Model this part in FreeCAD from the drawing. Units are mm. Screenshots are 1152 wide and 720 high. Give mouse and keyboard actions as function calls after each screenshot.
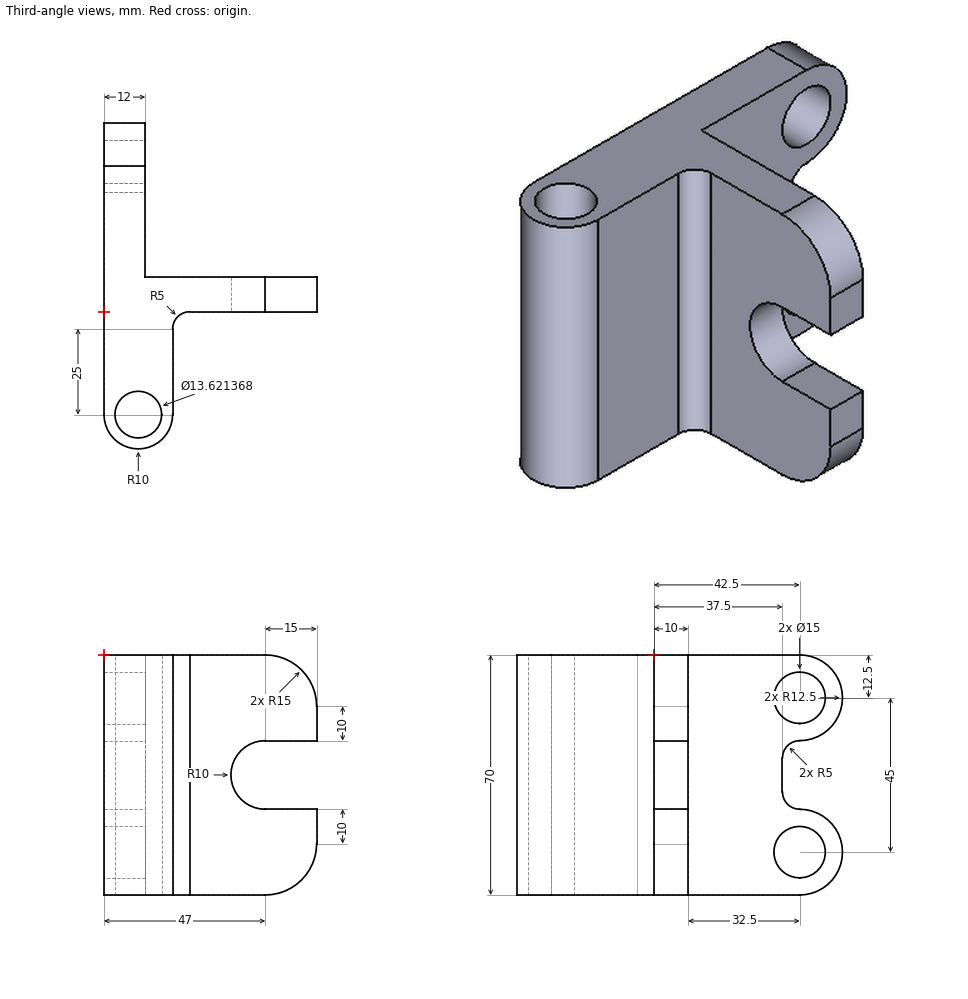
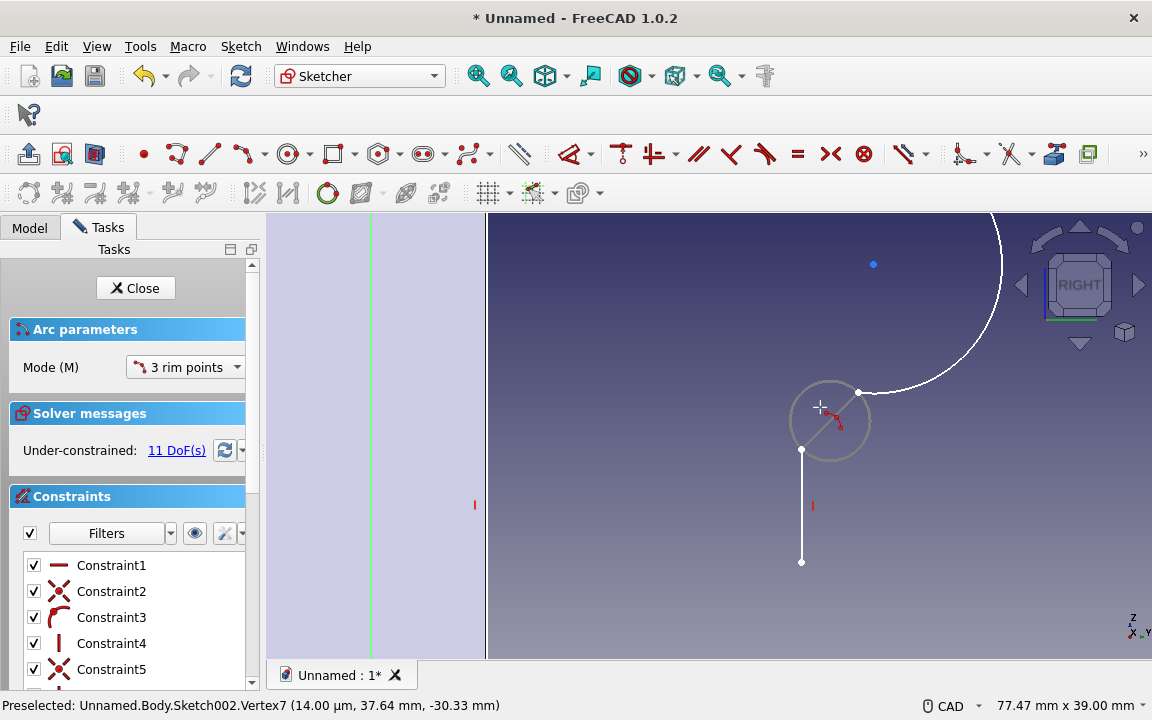
click(817, 405)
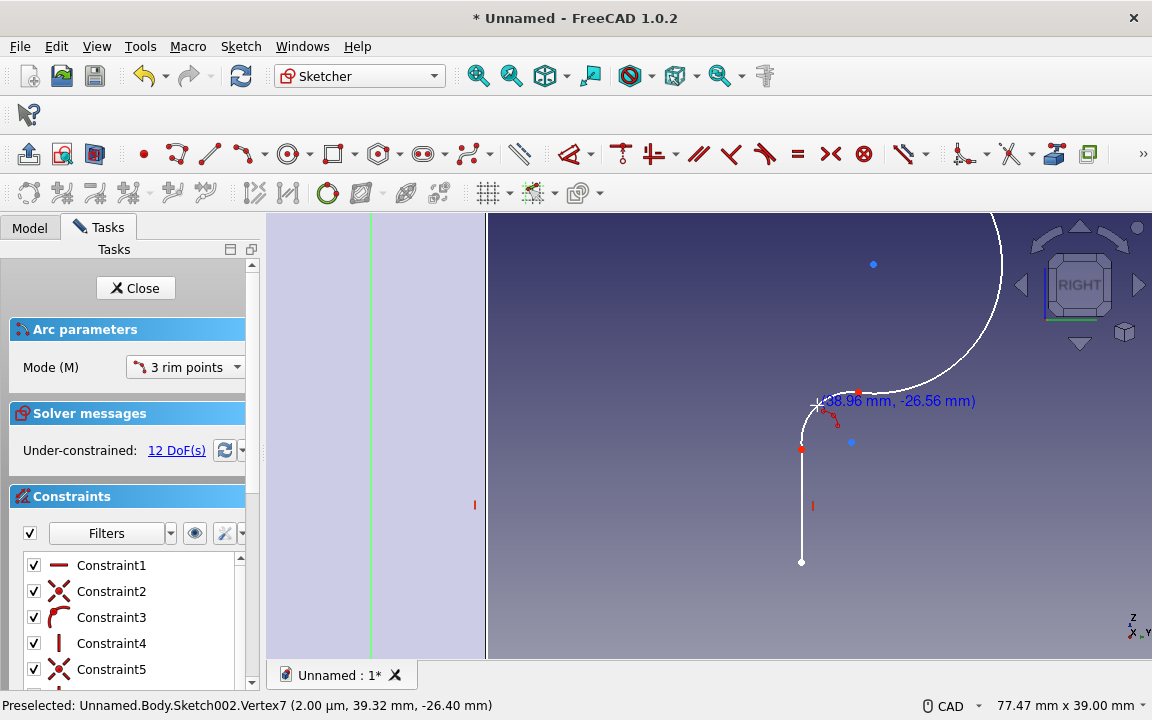
click(802, 562)
click(858, 617)
click(817, 600)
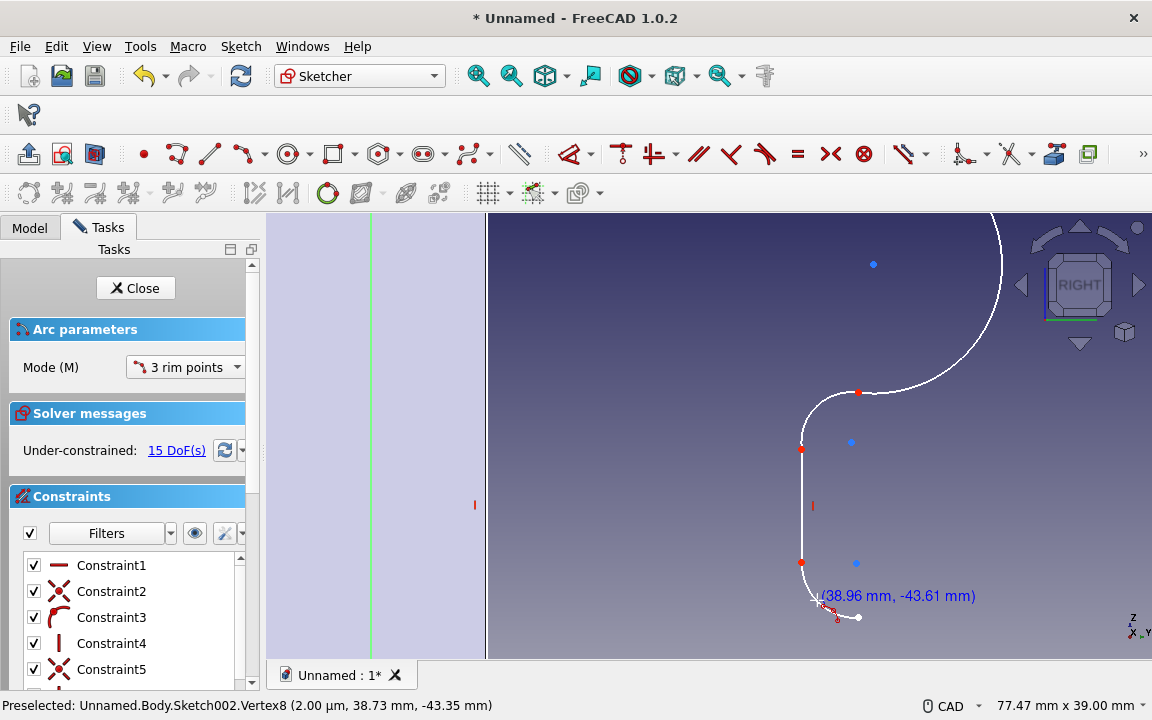
click(858, 618)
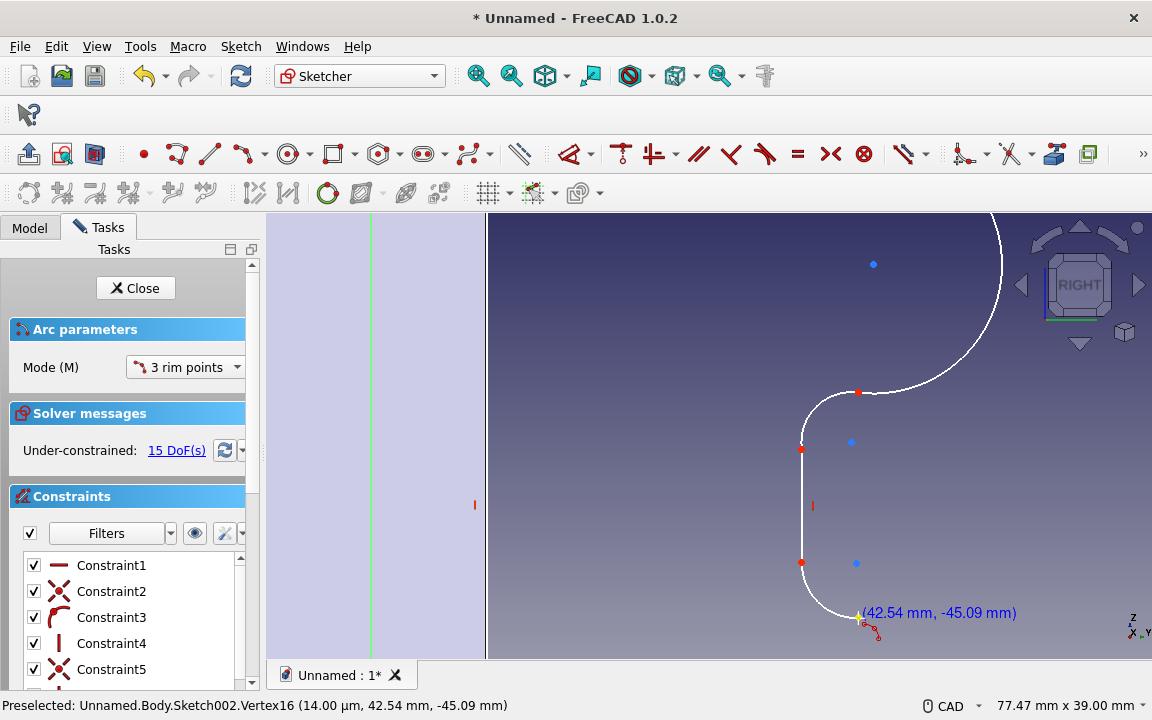
scroll(614, 397, down, 5)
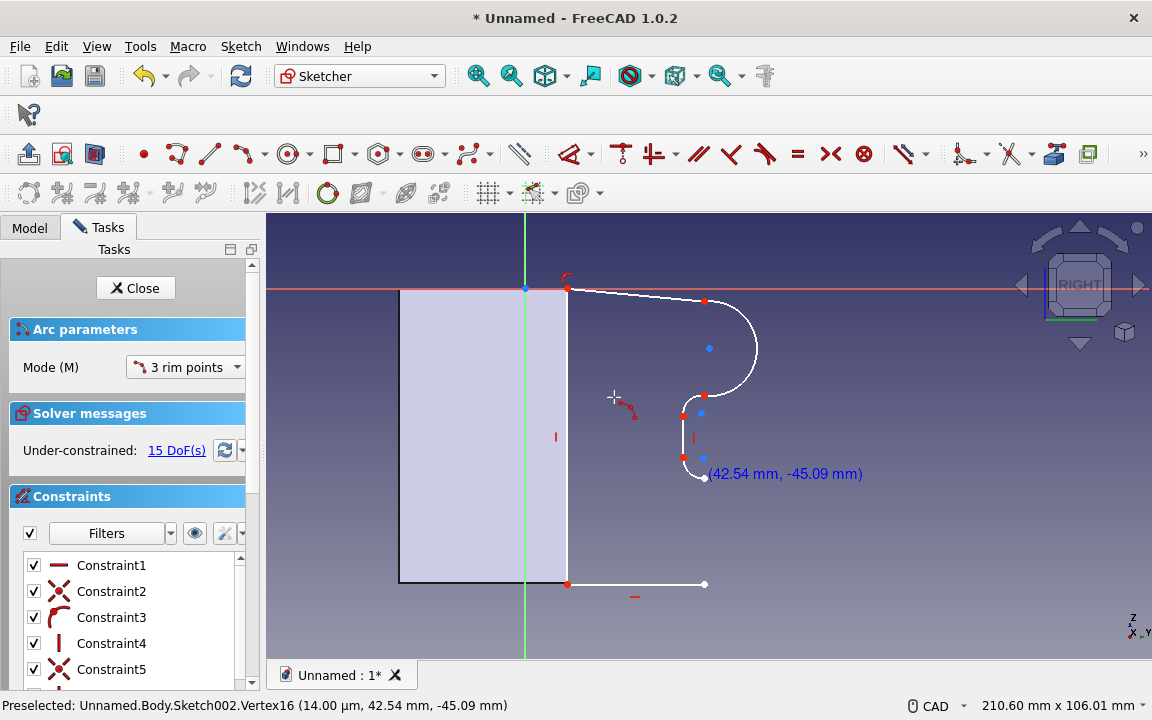
click(704, 585)
click(756, 531)
key(Escape)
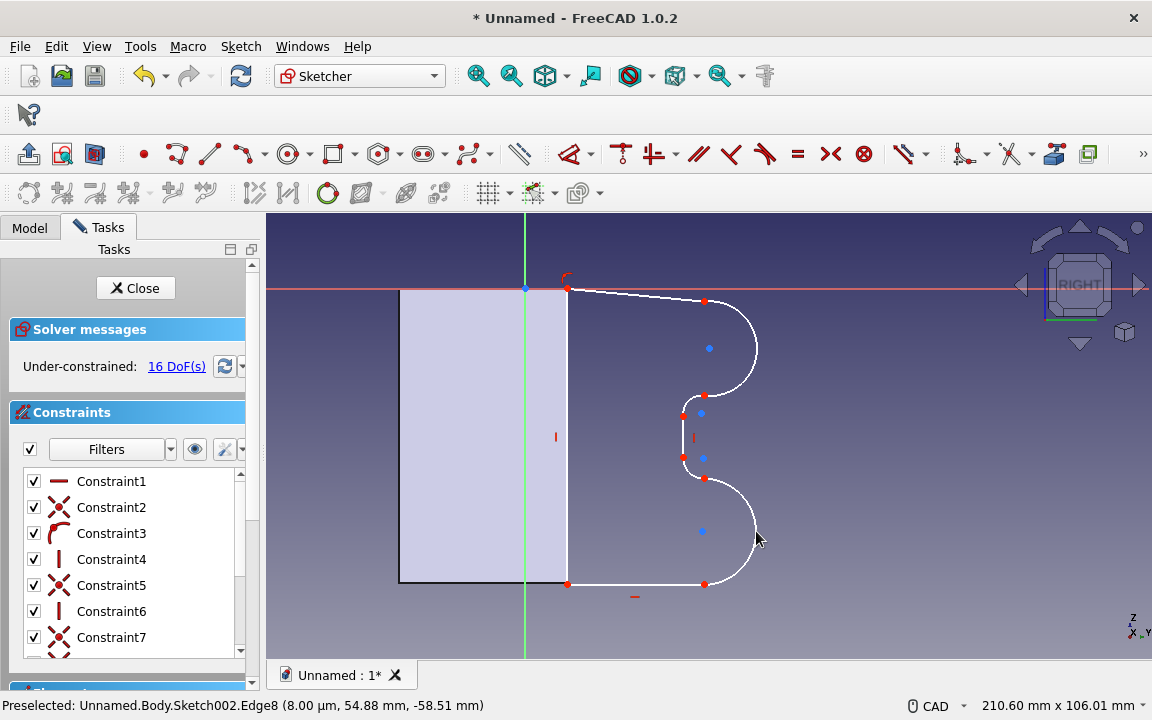
click(663, 585)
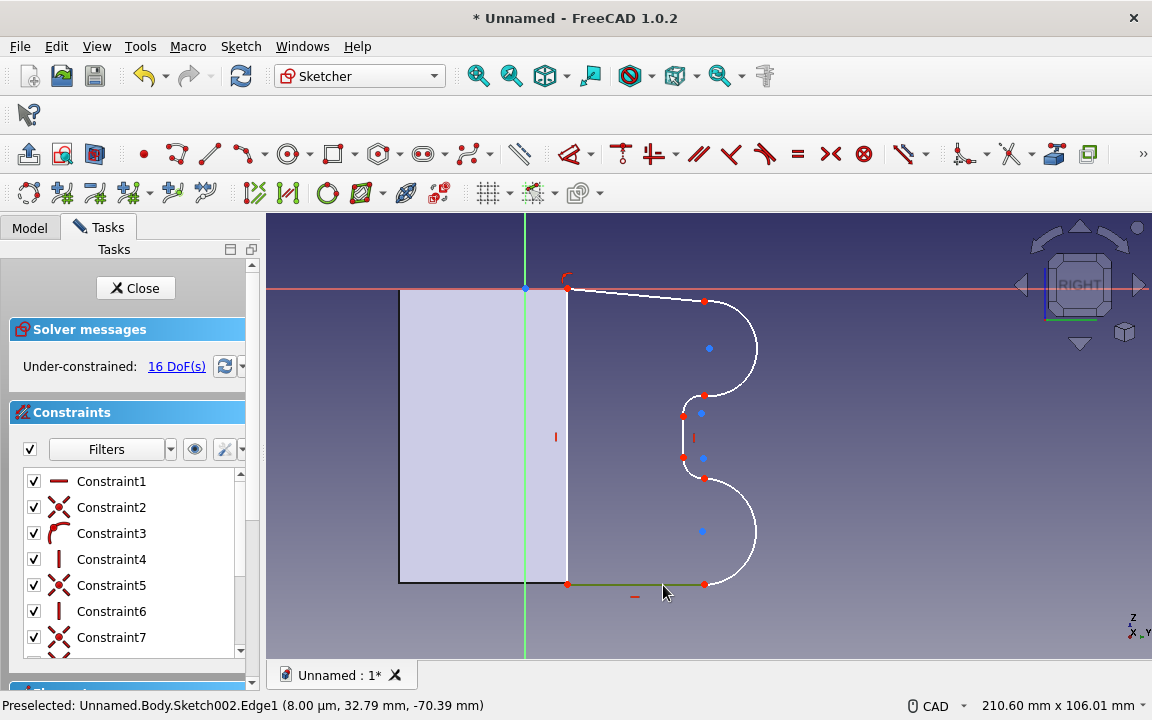
click(746, 563)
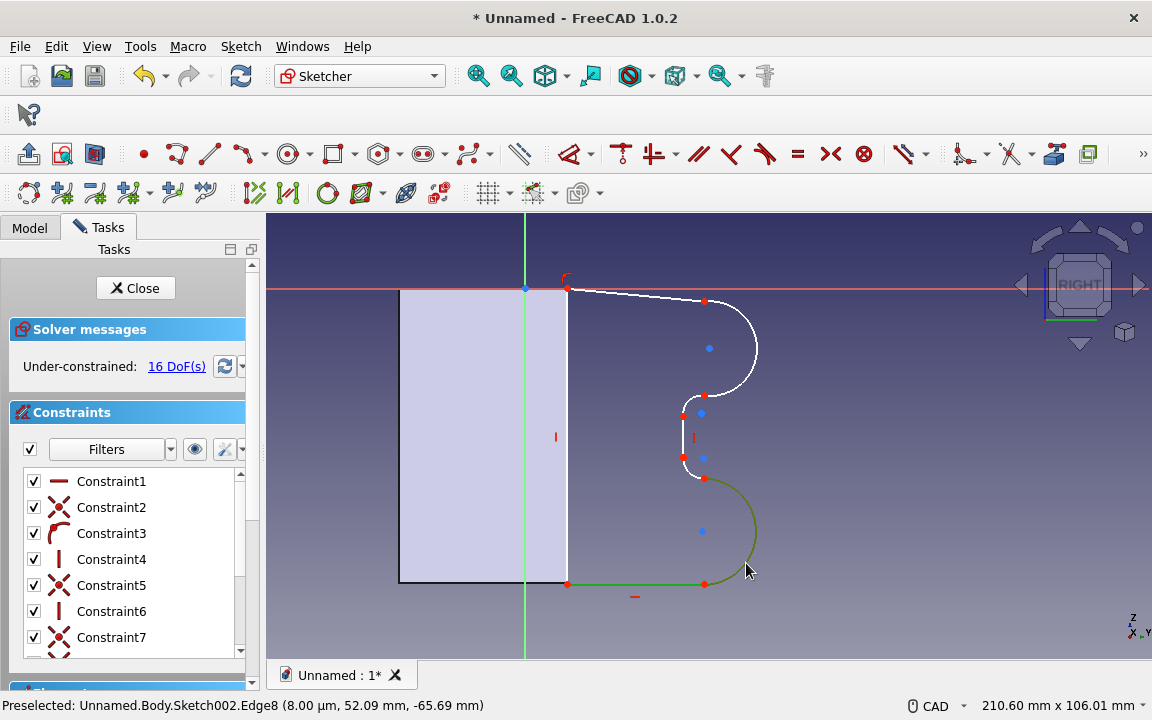
click(765, 154)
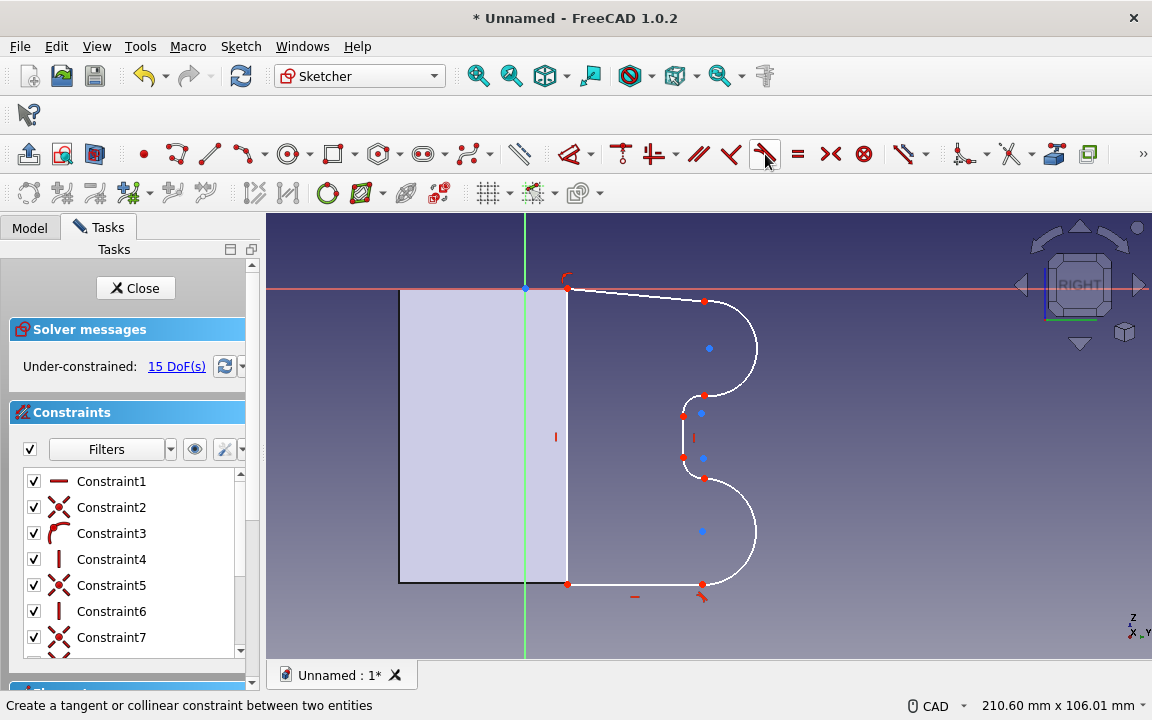
click(608, 293)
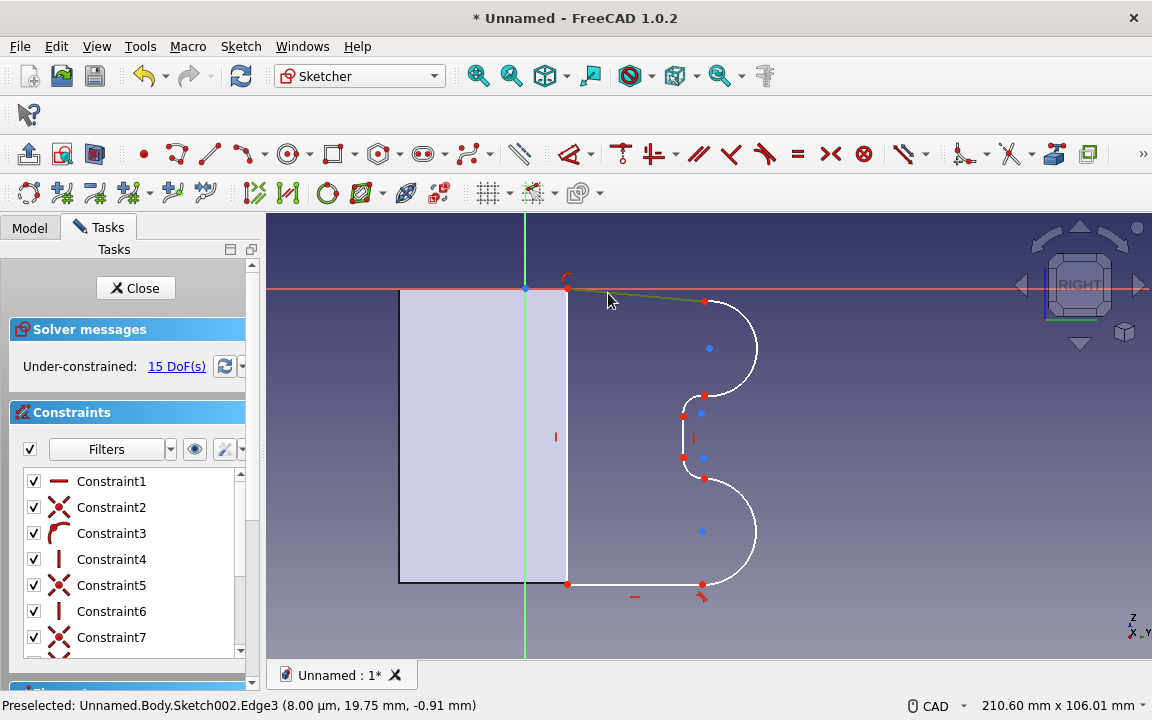
click(747, 378)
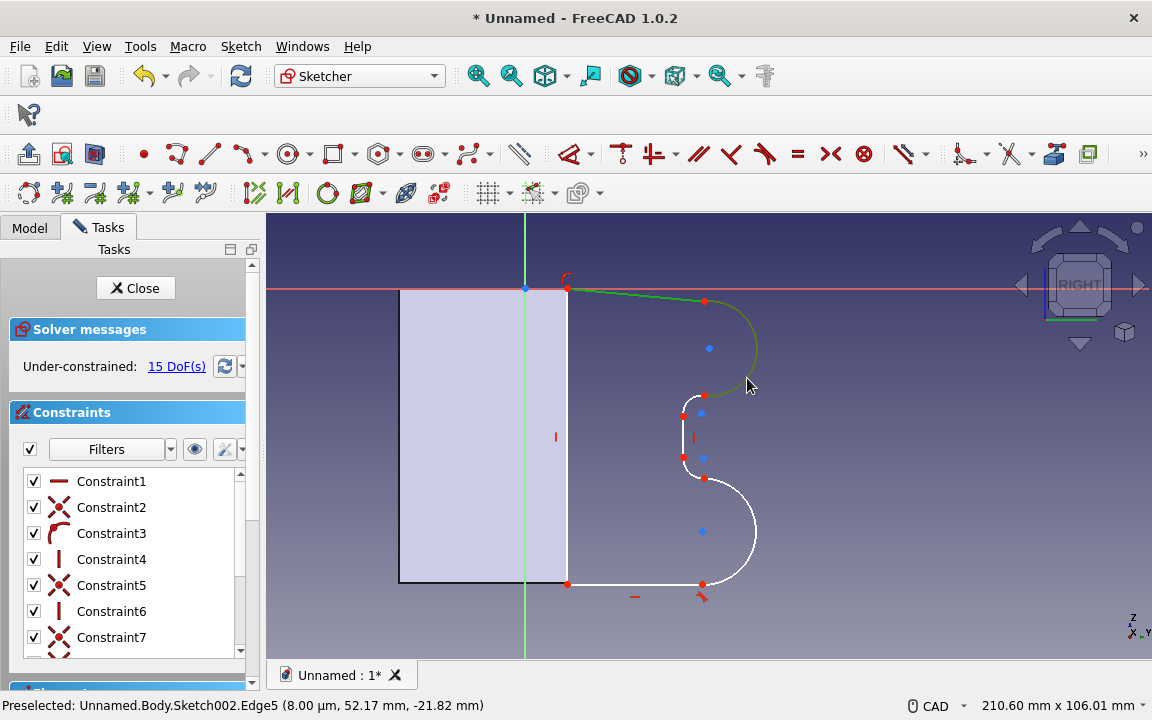
click(765, 154)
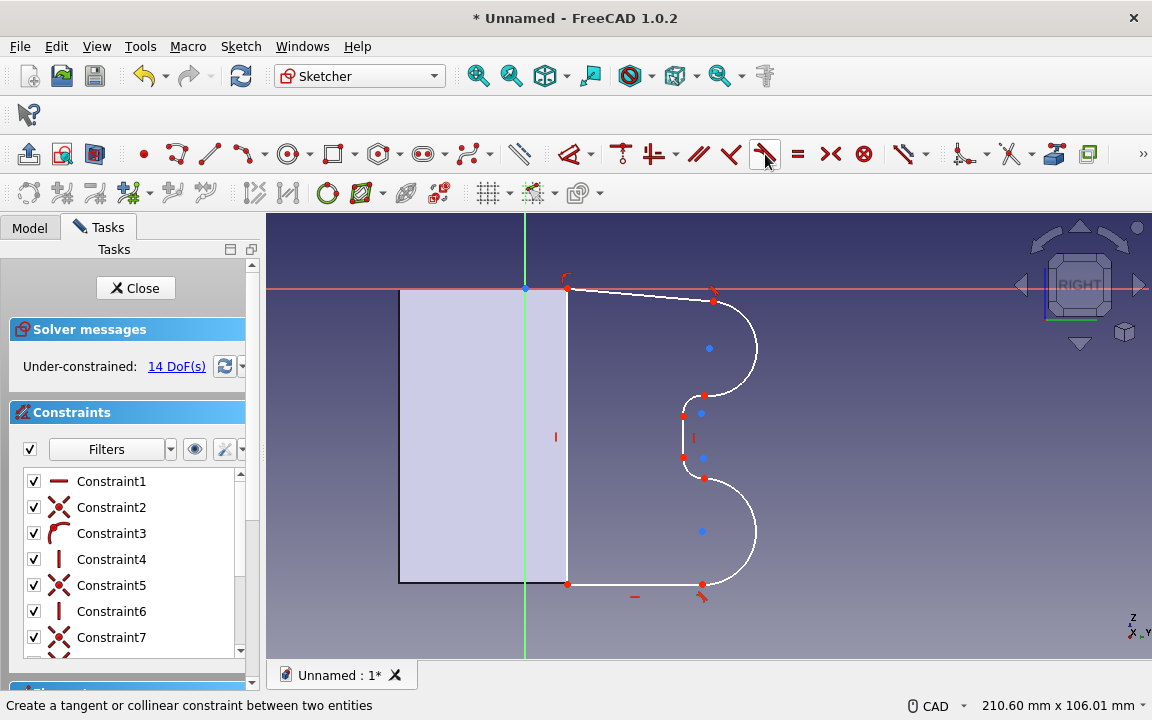
click(683, 429)